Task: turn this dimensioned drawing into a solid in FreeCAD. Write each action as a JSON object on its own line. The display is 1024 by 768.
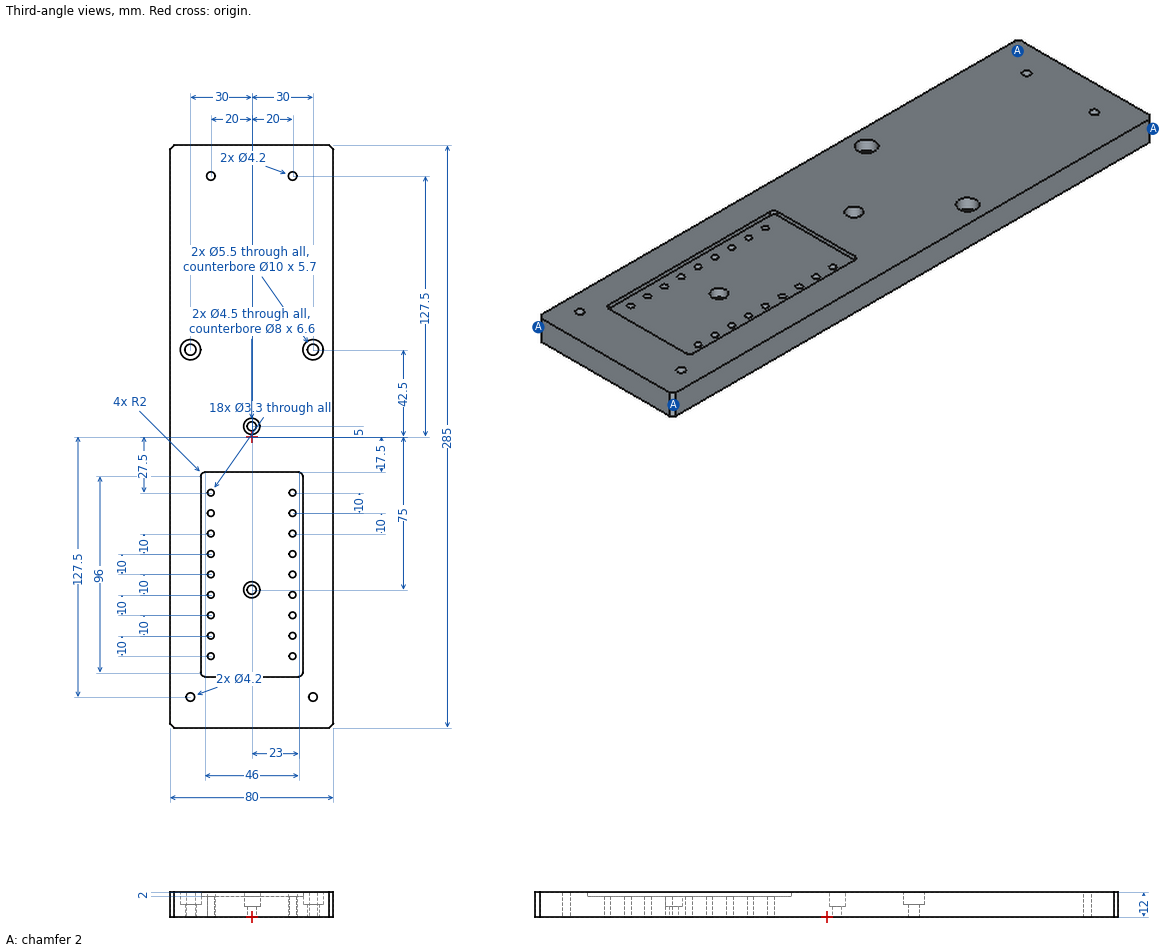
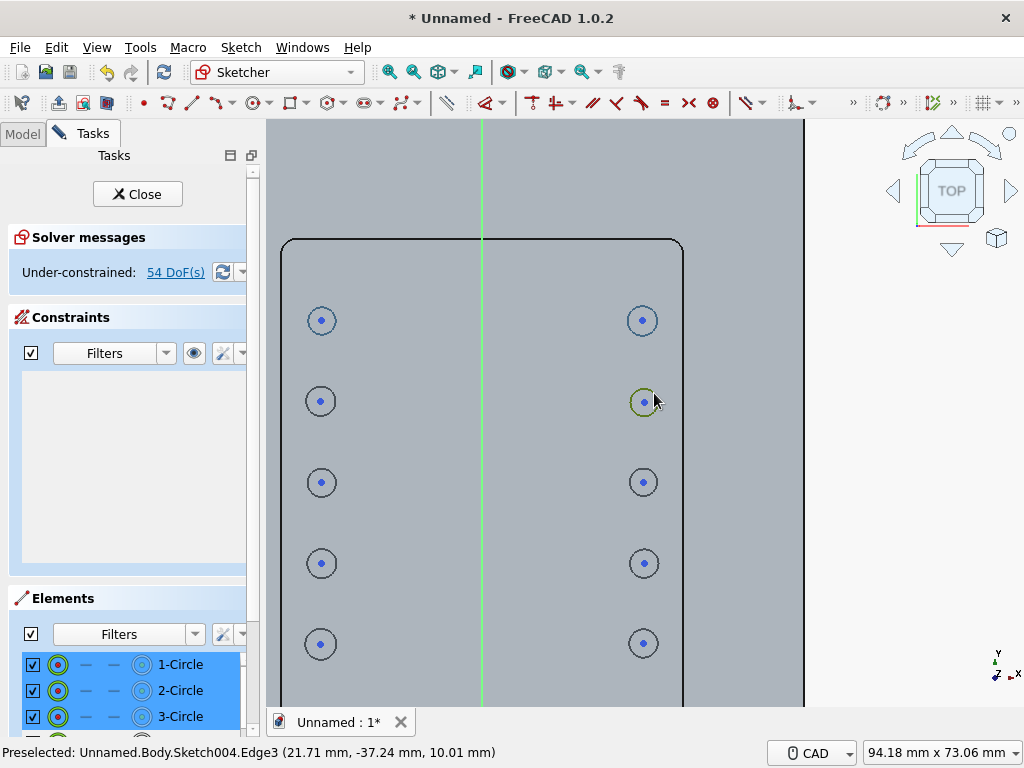
{"action": "left_click", "coordinate": [653, 472]}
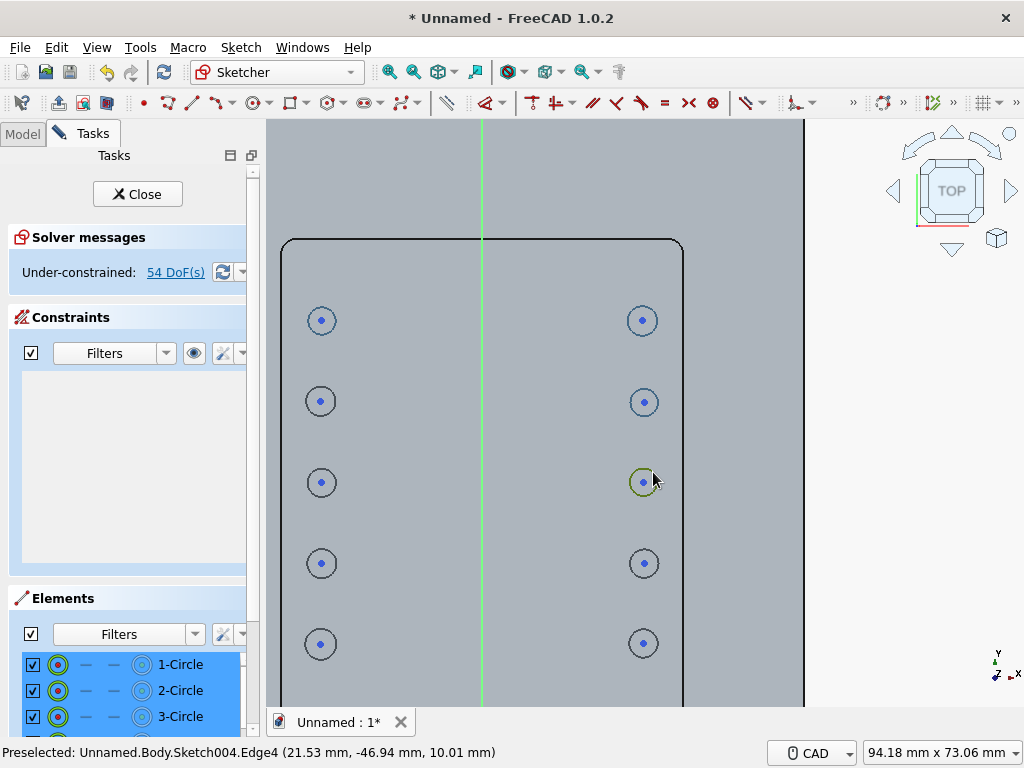
{"action": "left_click", "coordinate": [331, 391]}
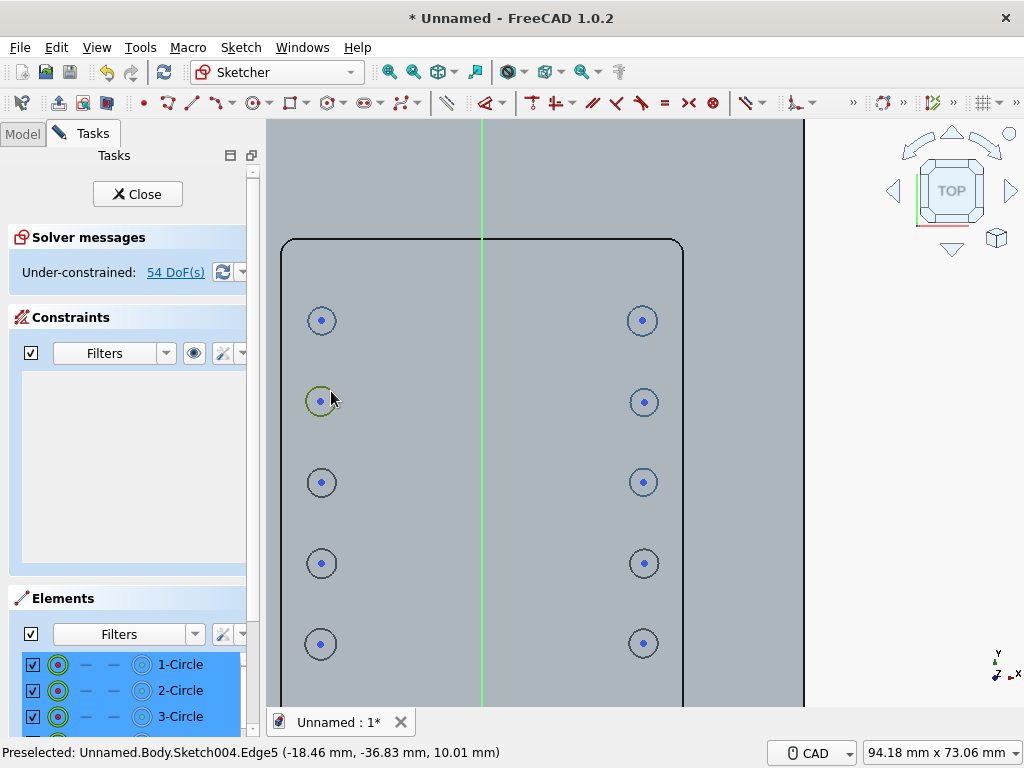
{"action": "left_click", "coordinate": [332, 473]}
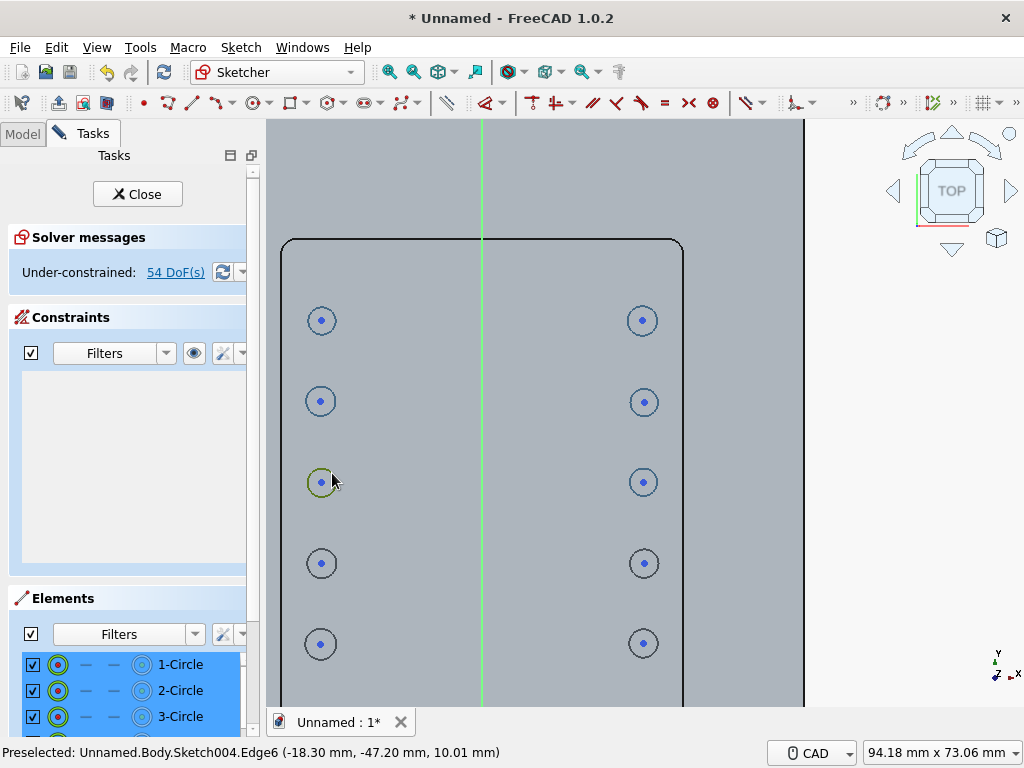
{"action": "left_click", "coordinate": [332, 553]}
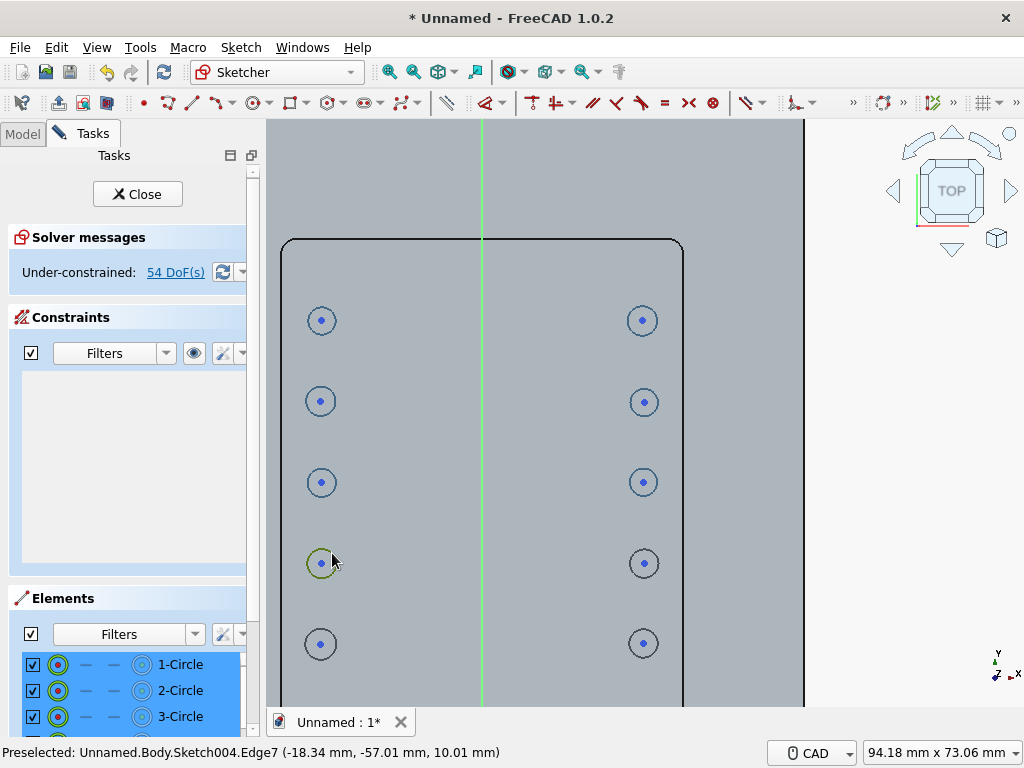
{"action": "left_click", "coordinate": [654, 554]}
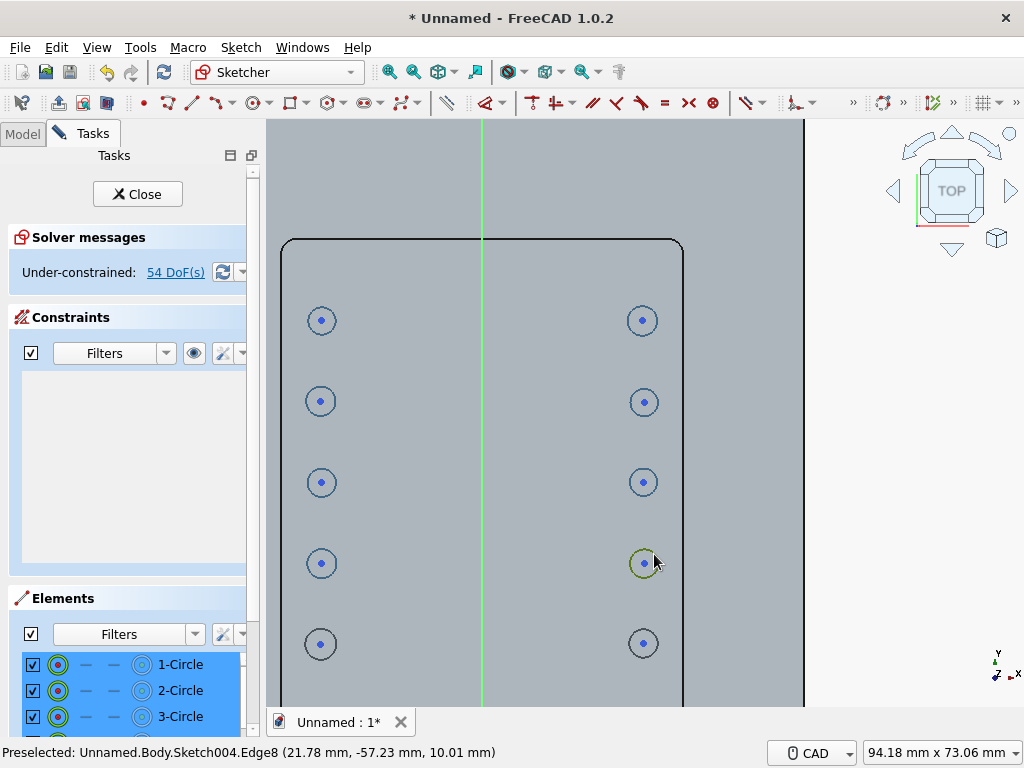
{"action": "left_click", "coordinate": [332, 633]}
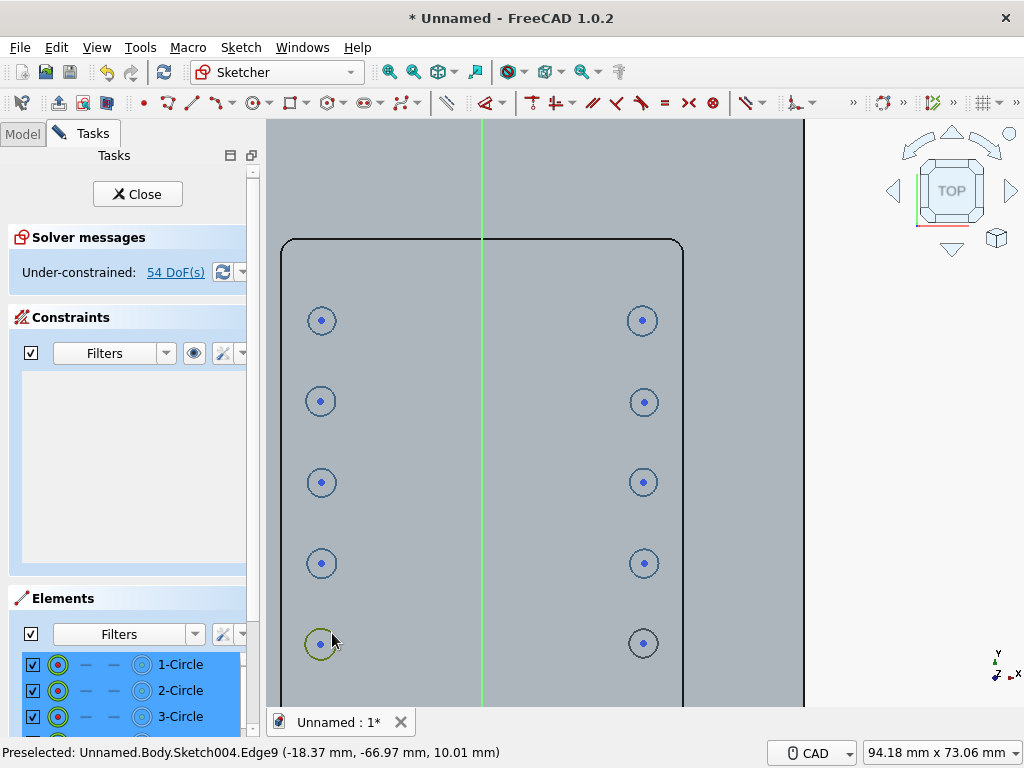
{"action": "left_click", "coordinate": [653, 633]}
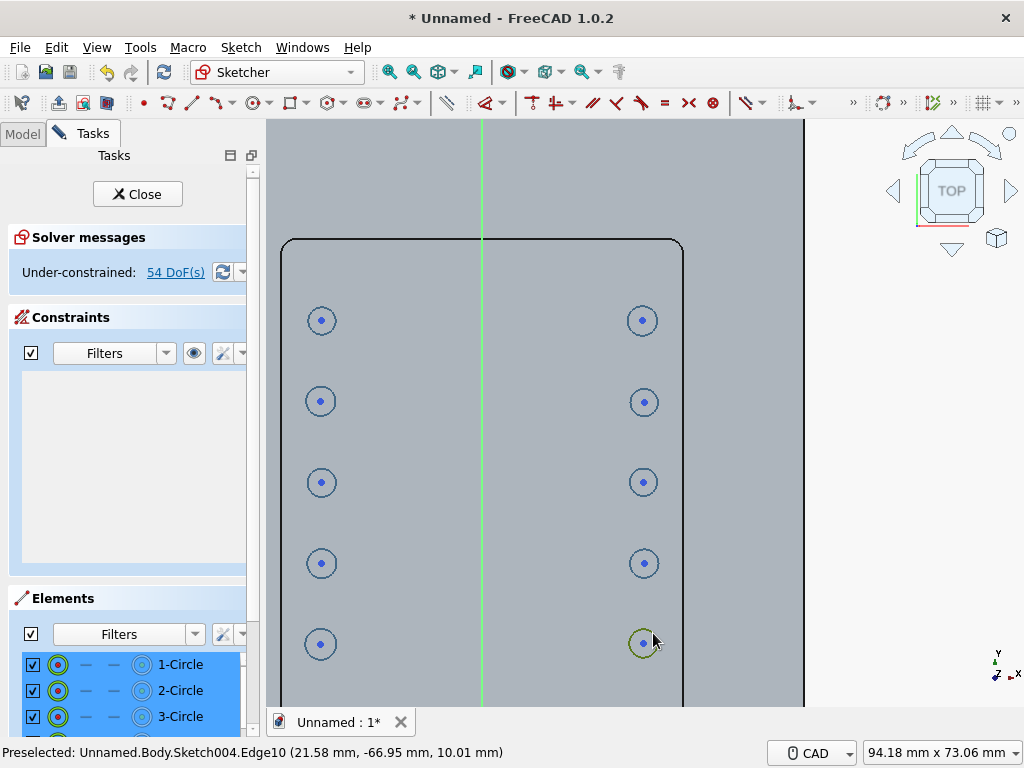
{"action": "scroll", "coordinate": [653, 312], "scroll_direction": "down", "scroll_amount": 4}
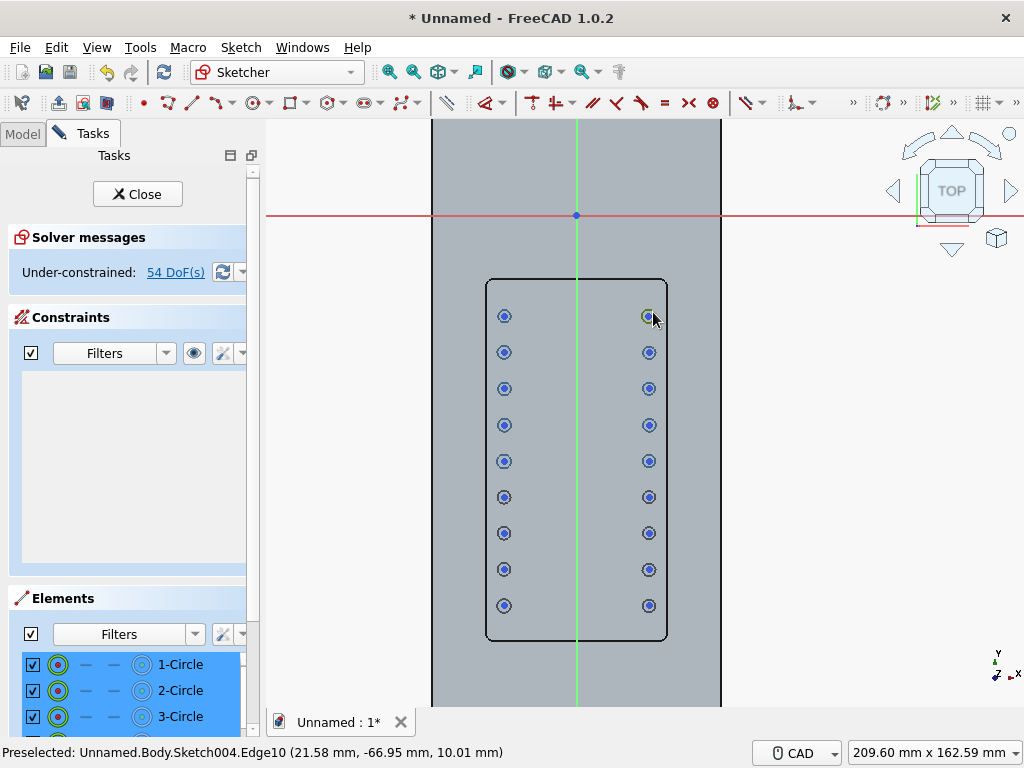
{"action": "scroll", "coordinate": [509, 493], "scroll_direction": "up", "scroll_amount": 4}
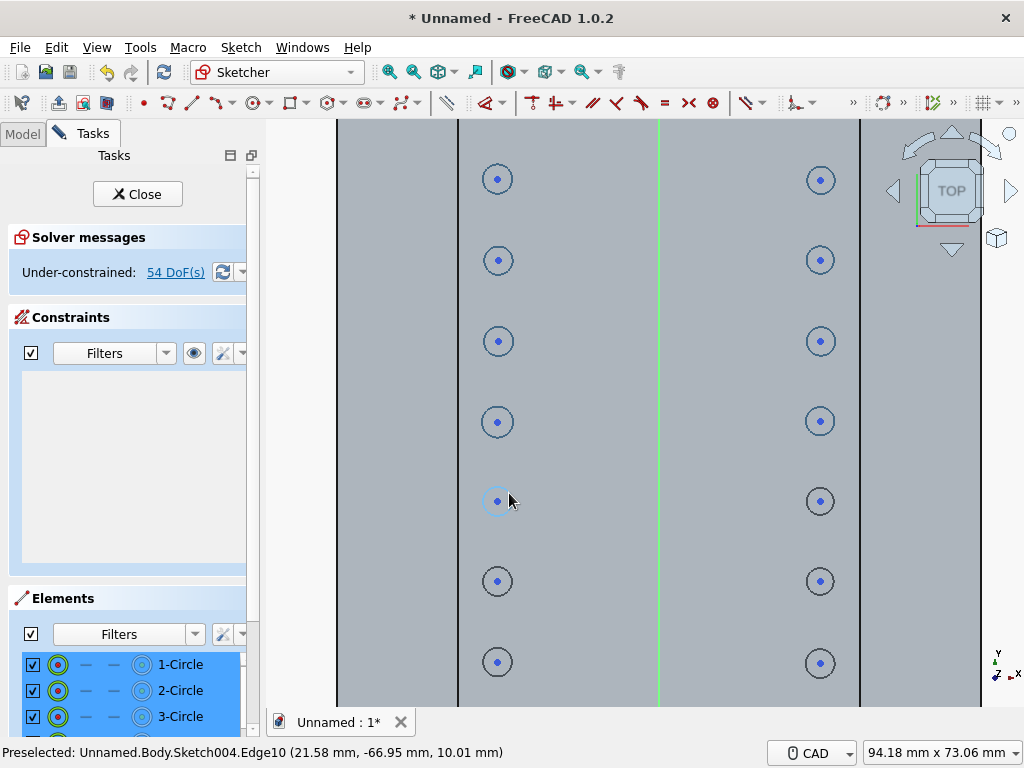
{"action": "left_click", "coordinate": [508, 491]}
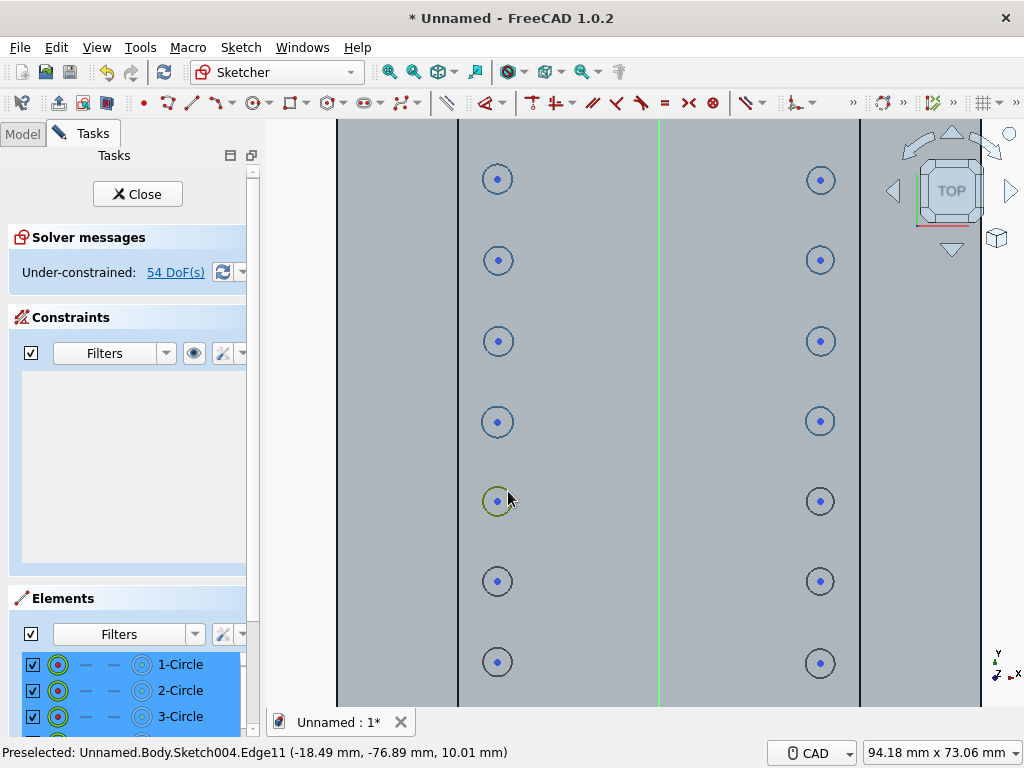
{"action": "left_click", "coordinate": [830, 492]}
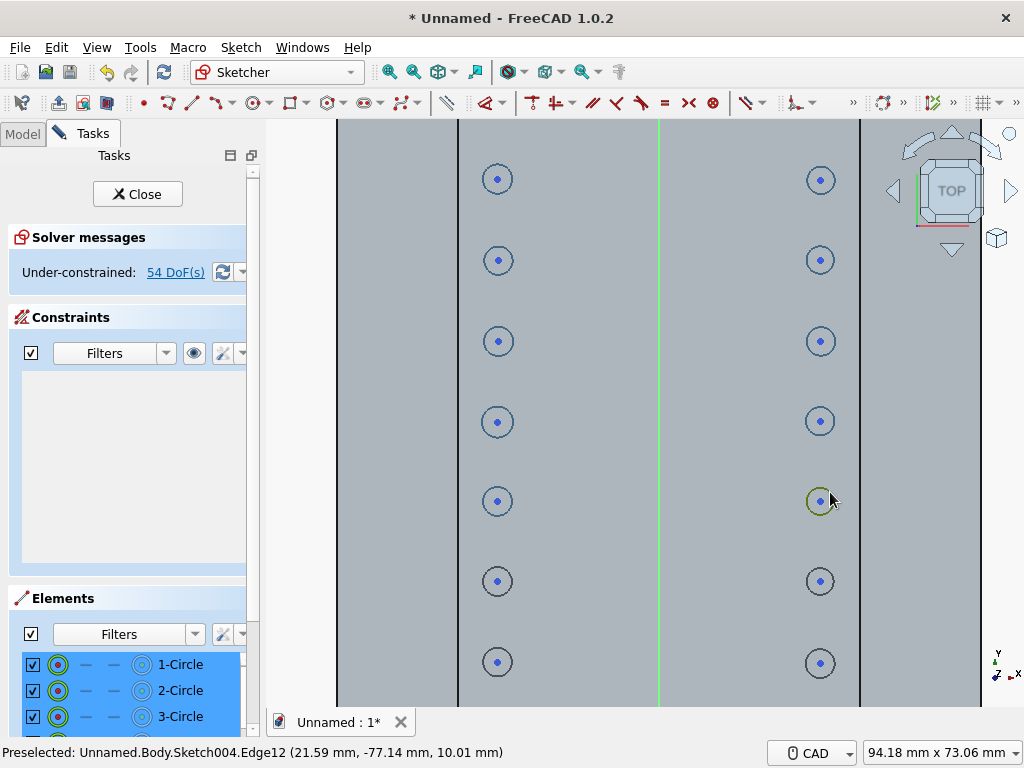
{"action": "left_click", "coordinate": [508, 571]}